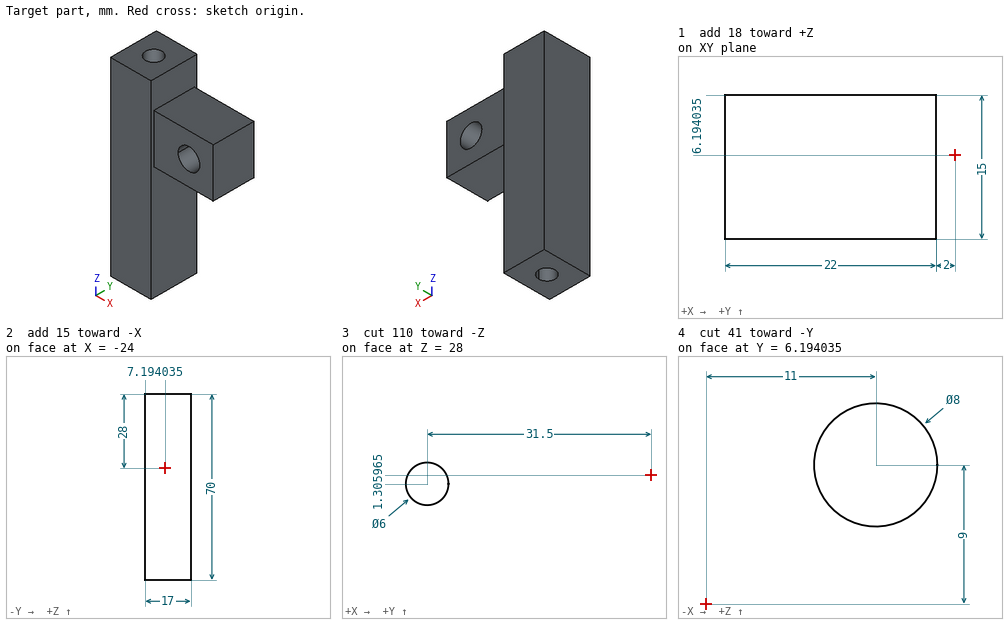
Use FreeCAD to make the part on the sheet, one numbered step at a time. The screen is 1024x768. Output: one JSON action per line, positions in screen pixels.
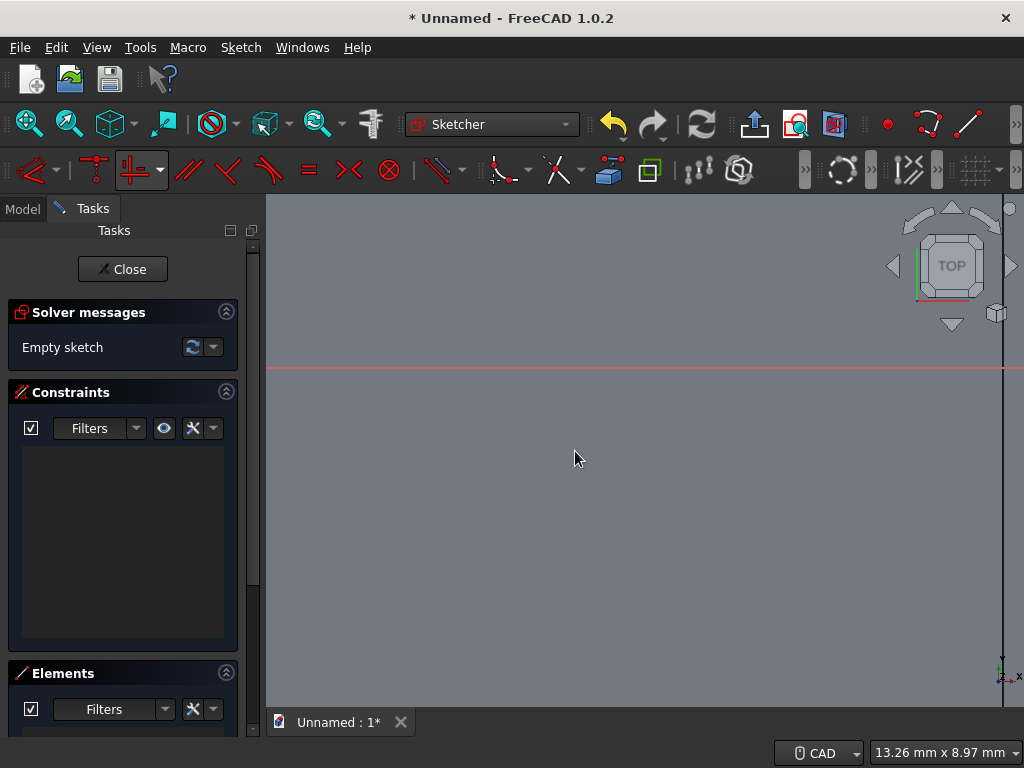
{"action": "key", "text": "g c"}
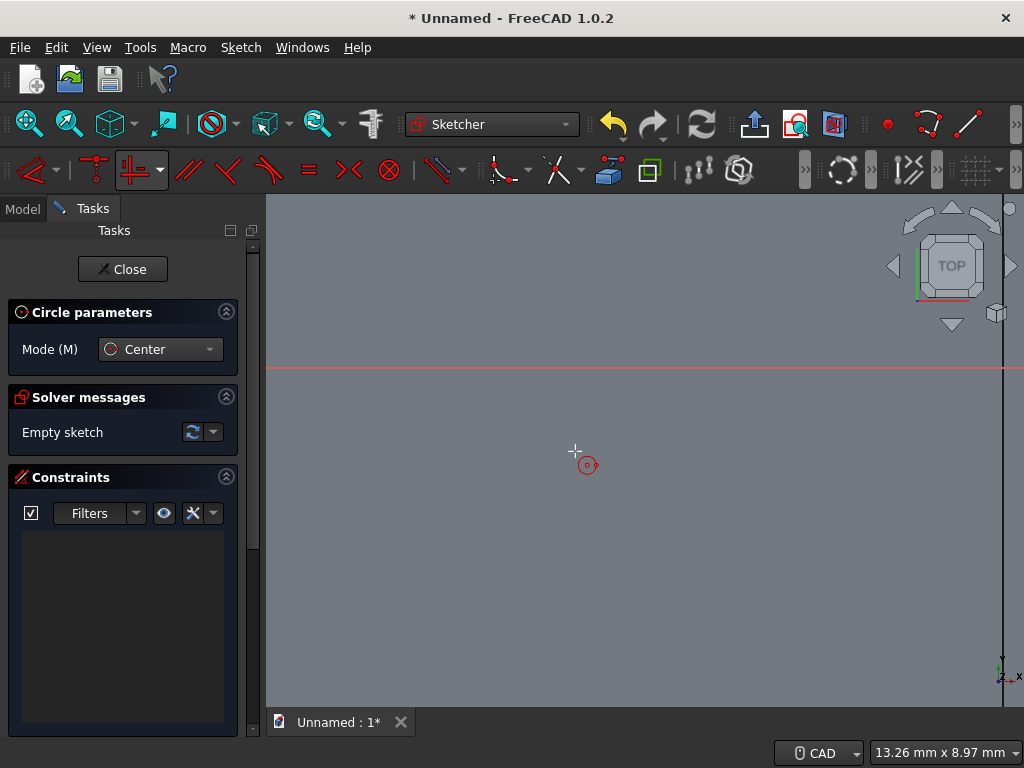
{"action": "left_click", "coordinate": [575, 442]}
{"action": "mouse_move", "coordinate": [696, 321]}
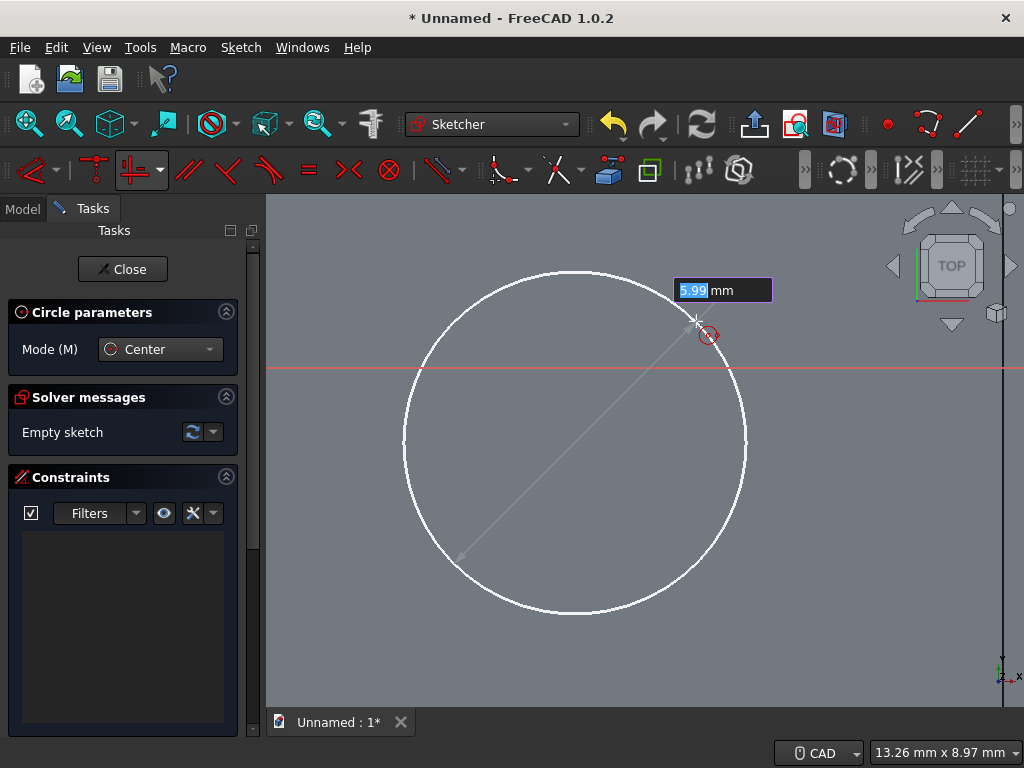
{"action": "type", "text": "6"}
{"action": "key", "text": "Return"}
{"action": "key", "text": "Escape"}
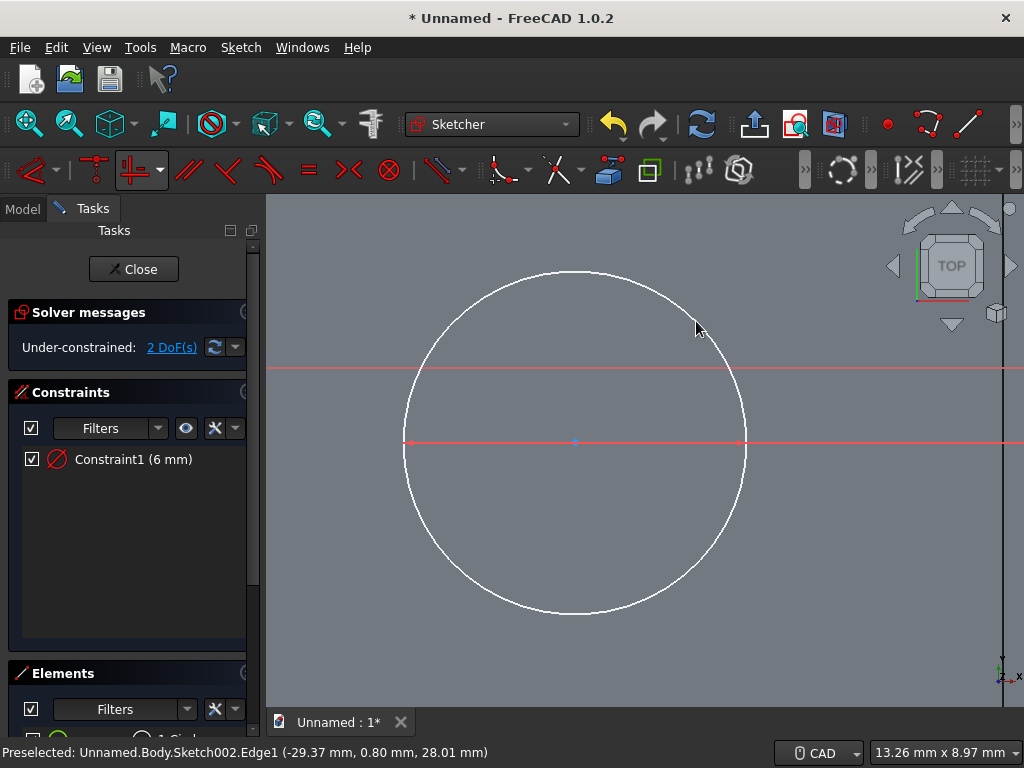
{"action": "left_click", "coordinate": [32, 170]}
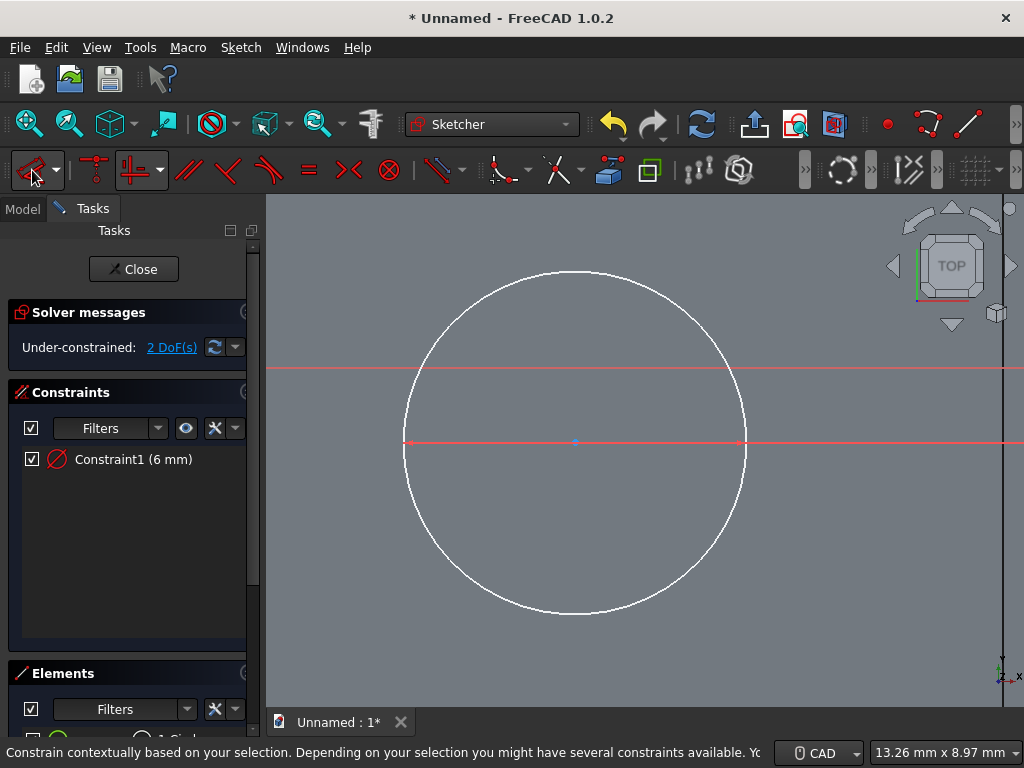
{"action": "left_click", "coordinate": [575, 443]}
{"action": "left_click", "coordinate": [652, 334]}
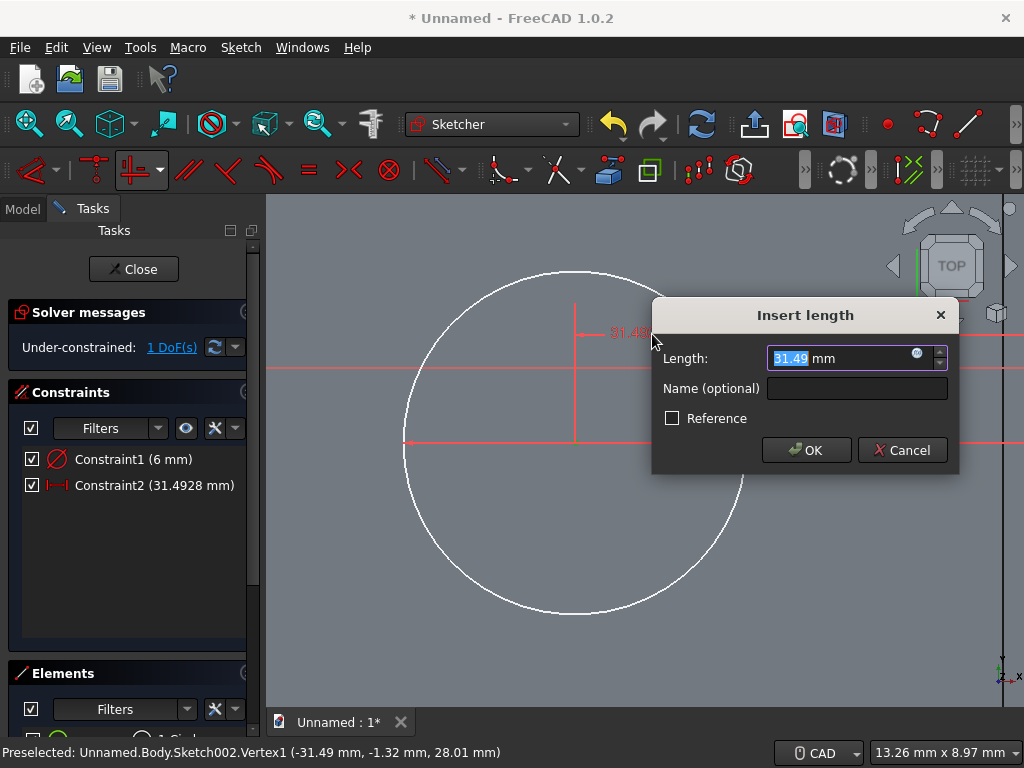
{"action": "type", "text": "31.5"}
{"action": "key", "text": "Return"}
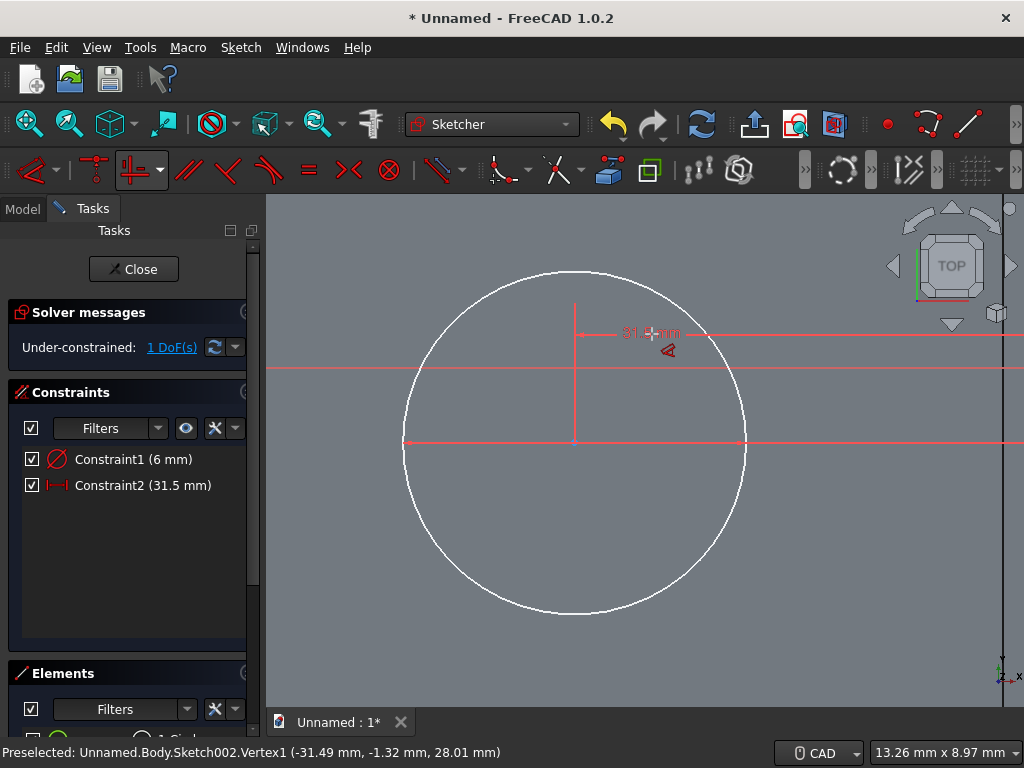
{"action": "left_click", "coordinate": [575, 443]}
{"action": "left_click", "coordinate": [541, 405]}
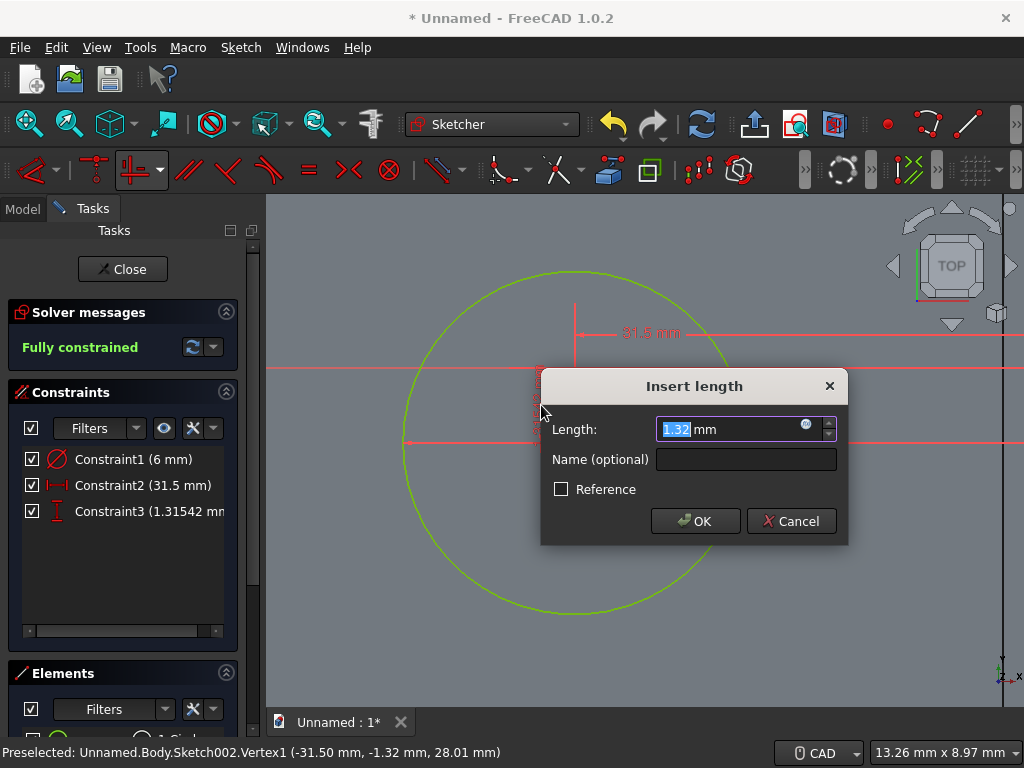
{"action": "type", "text": "1.305965"}
{"action": "key", "text": "Return"}
{"action": "key", "text": "Escape"}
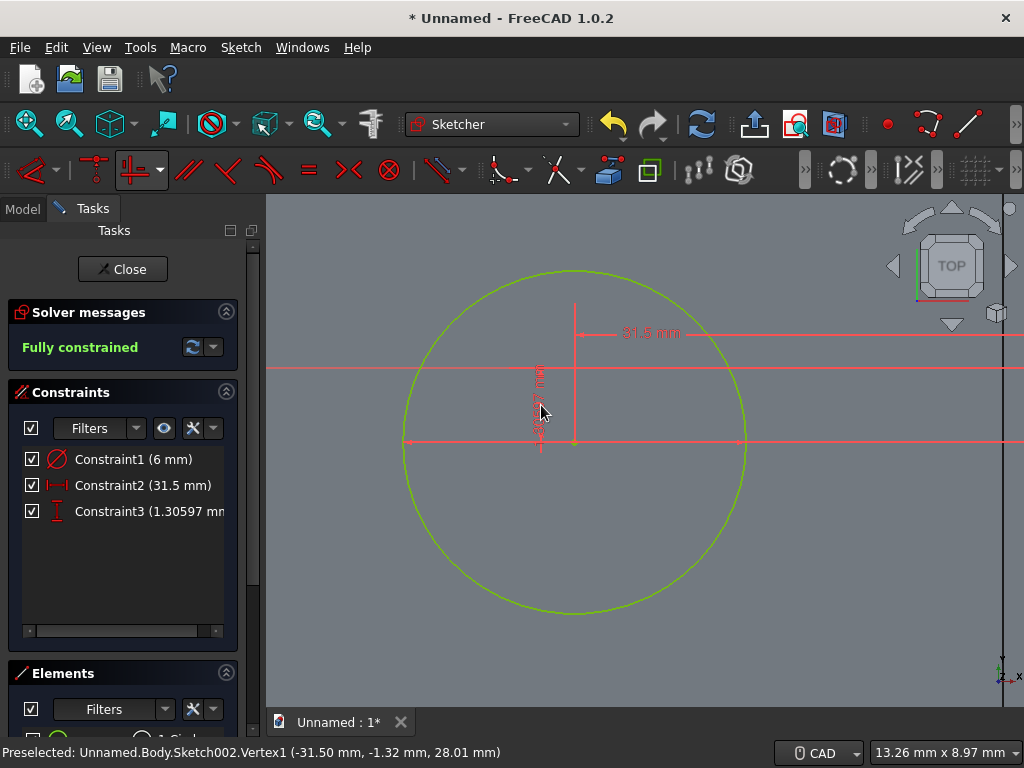
{"action": "left_click", "coordinate": [123, 269]}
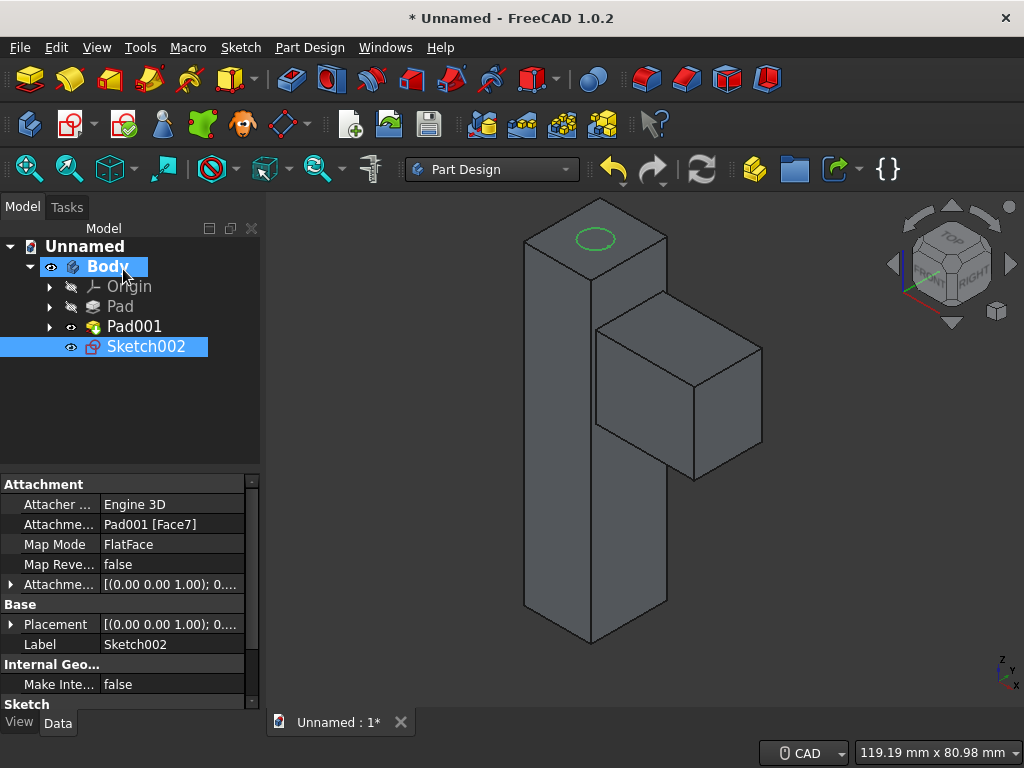
{"action": "left_click", "coordinate": [292, 80]}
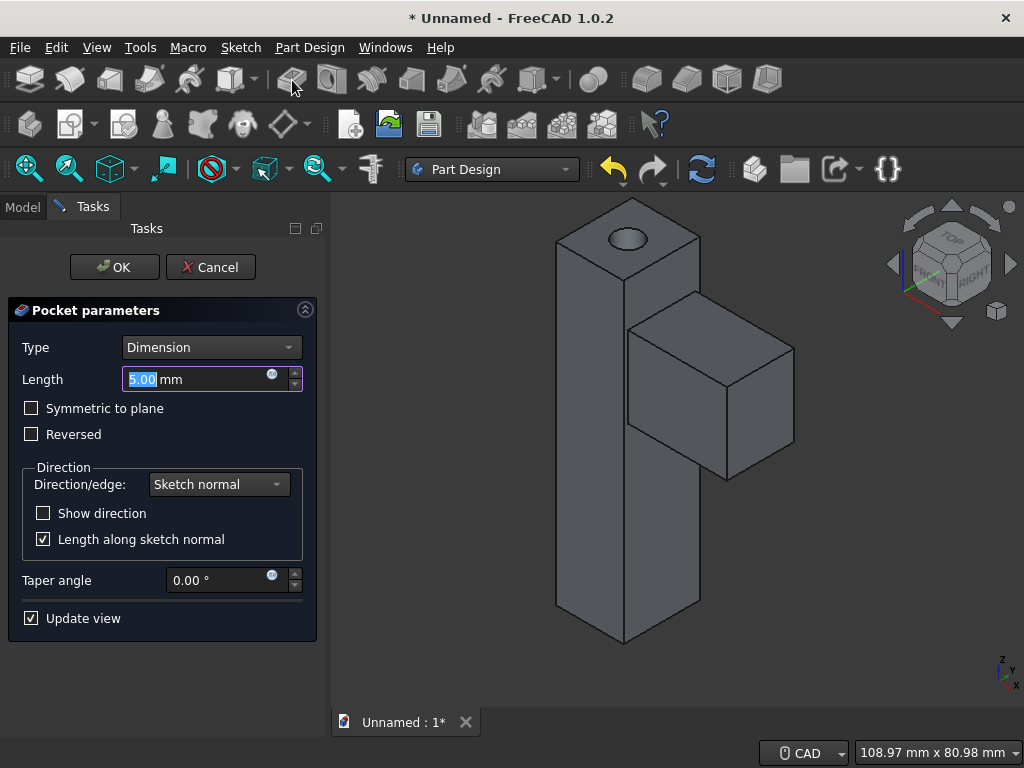
{"action": "type", "text": "110"}
{"action": "key", "text": "Tab"}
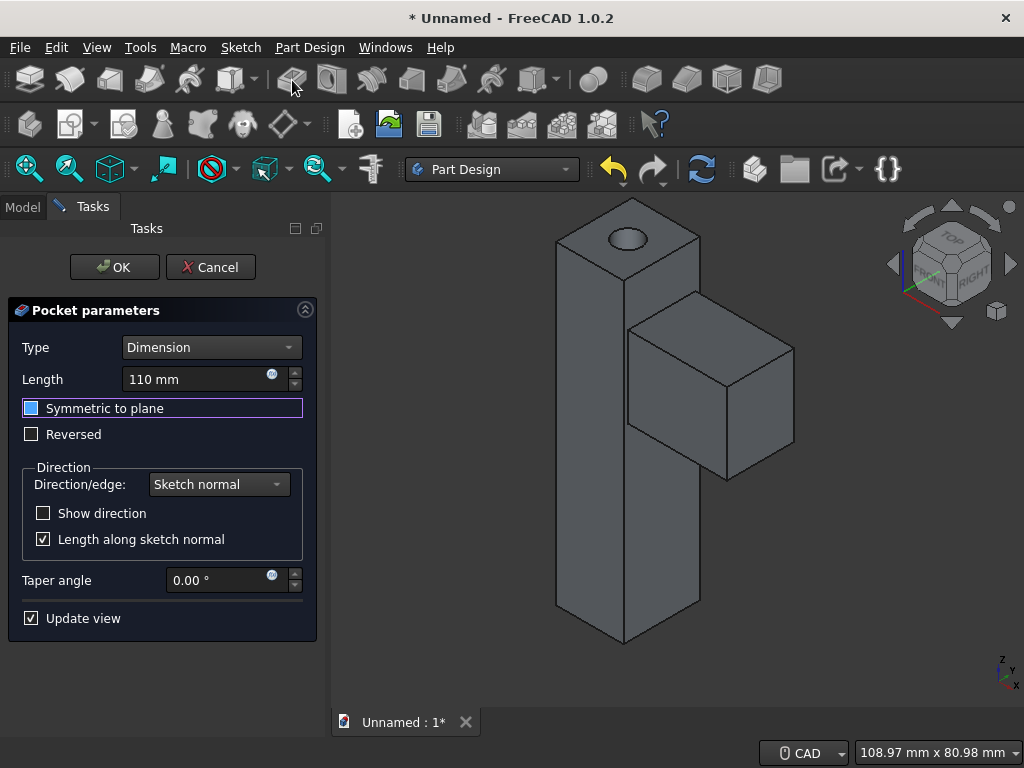
{"action": "left_click", "coordinate": [115, 267]}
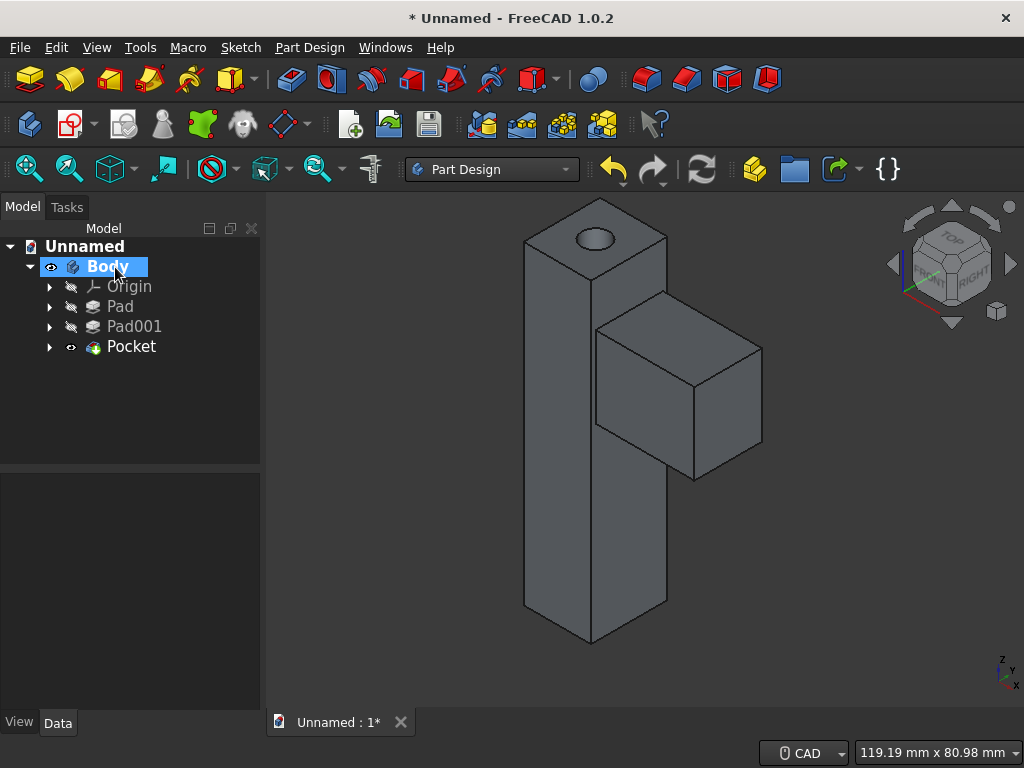
{"action": "key", "text": "4"}